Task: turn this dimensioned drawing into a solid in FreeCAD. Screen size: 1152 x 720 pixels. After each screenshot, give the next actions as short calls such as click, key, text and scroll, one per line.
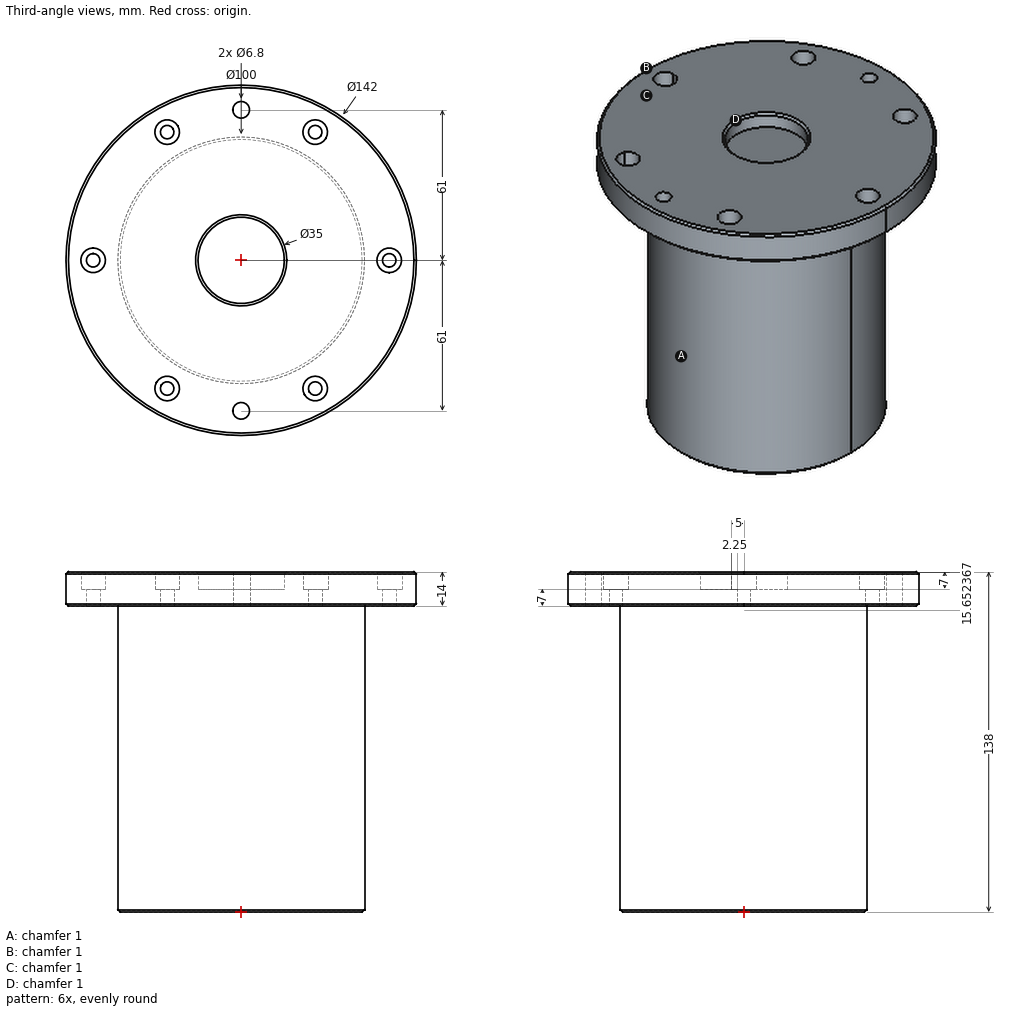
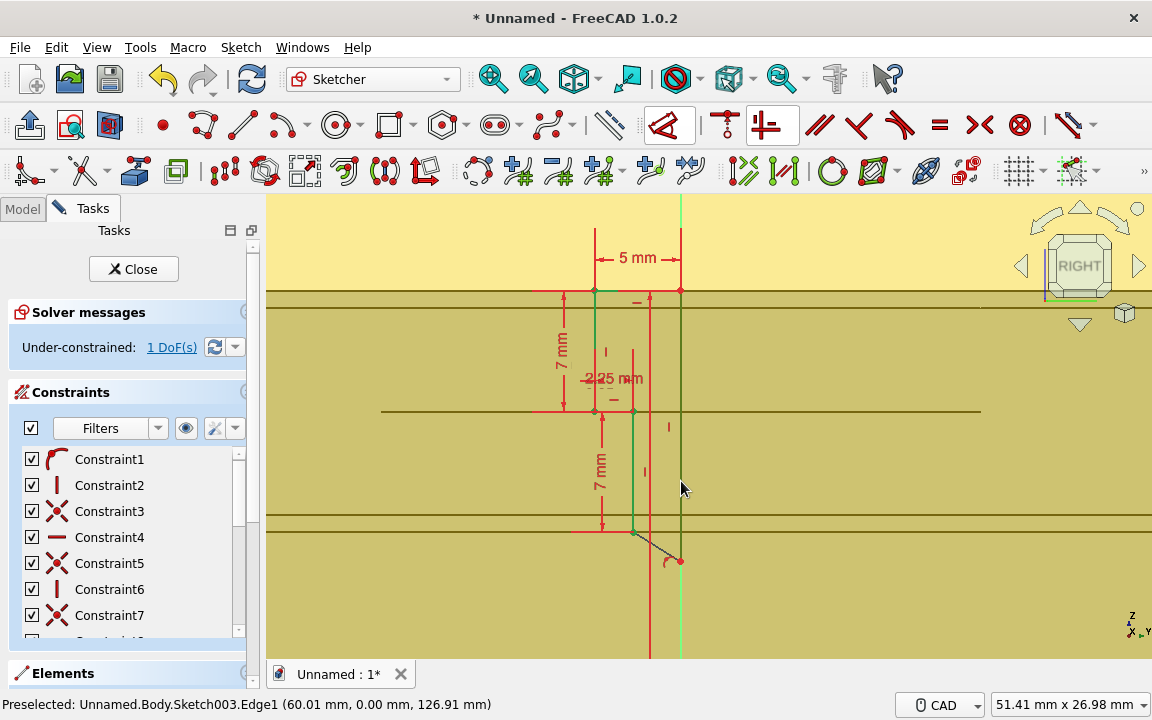
key(i)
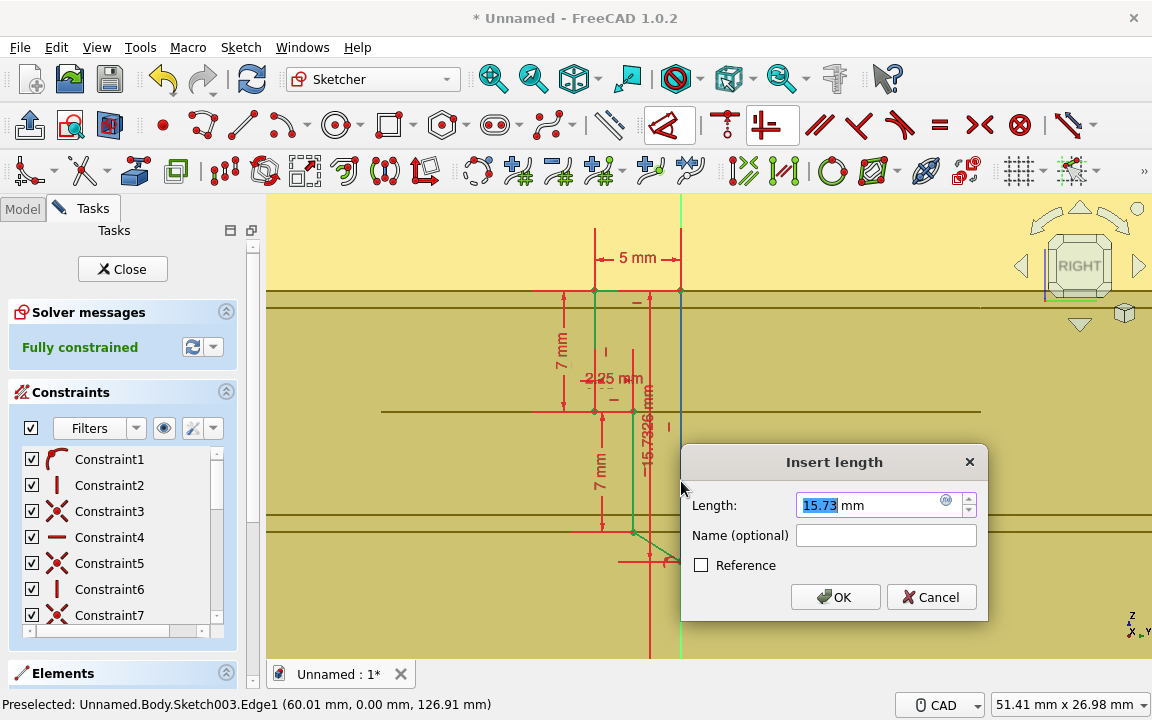
text(15.652367)
key(Return)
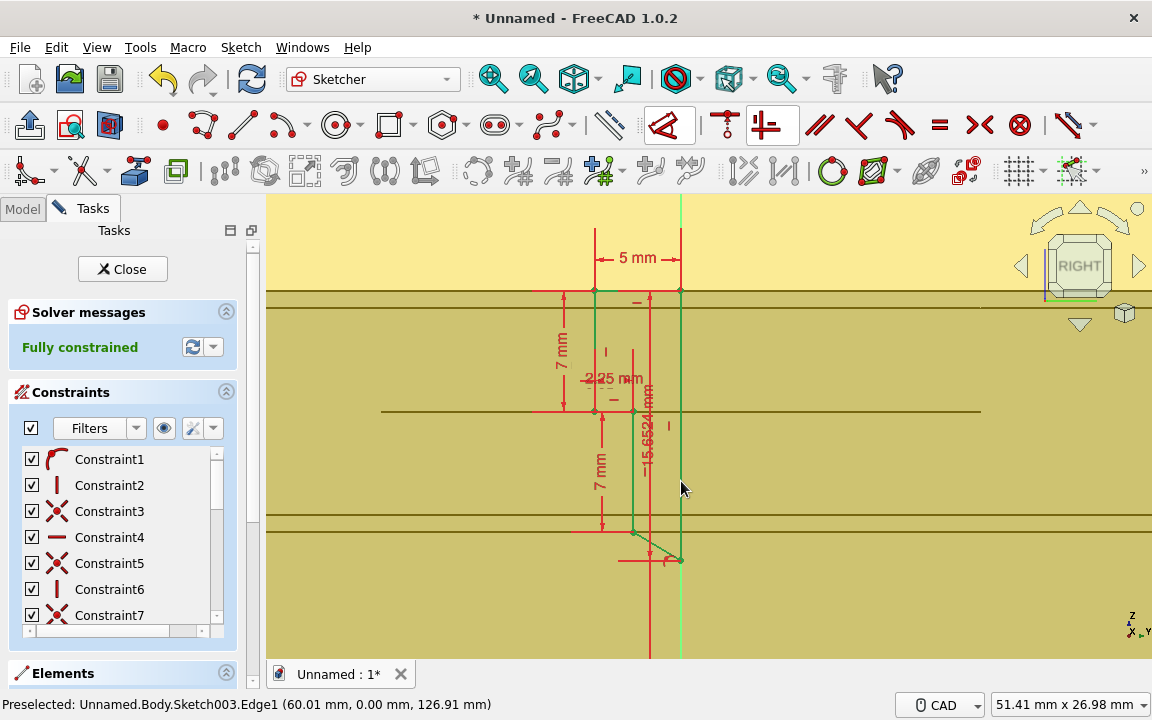
click(123, 269)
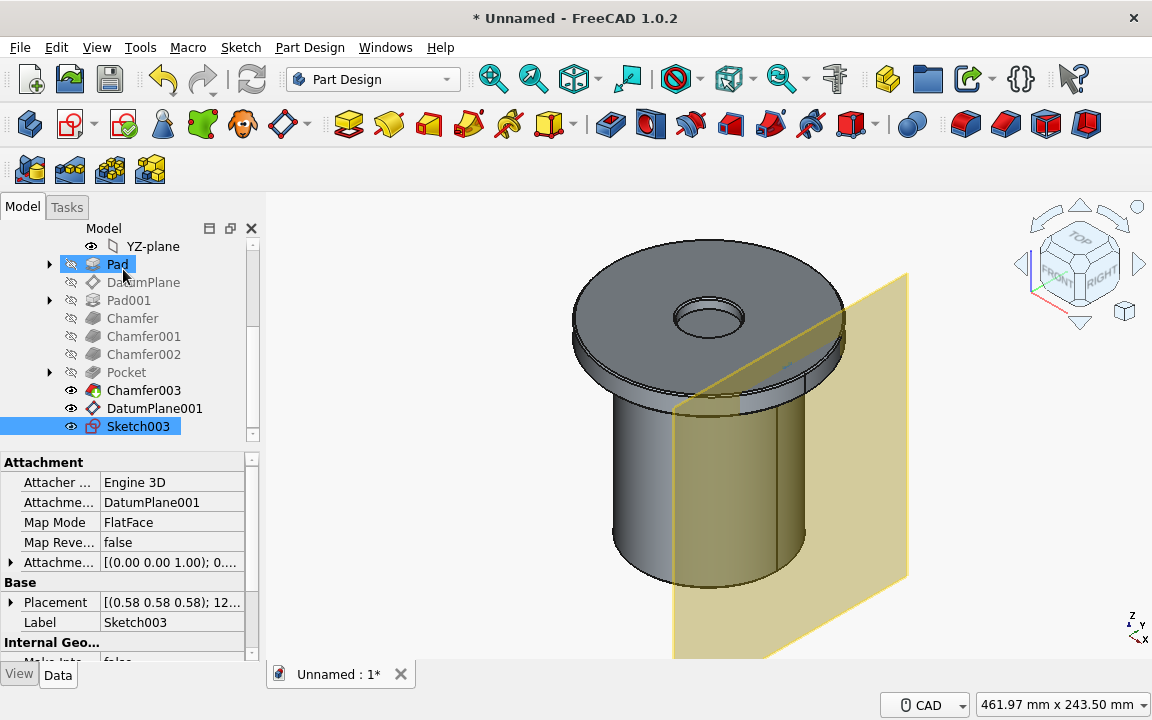
click(692, 124)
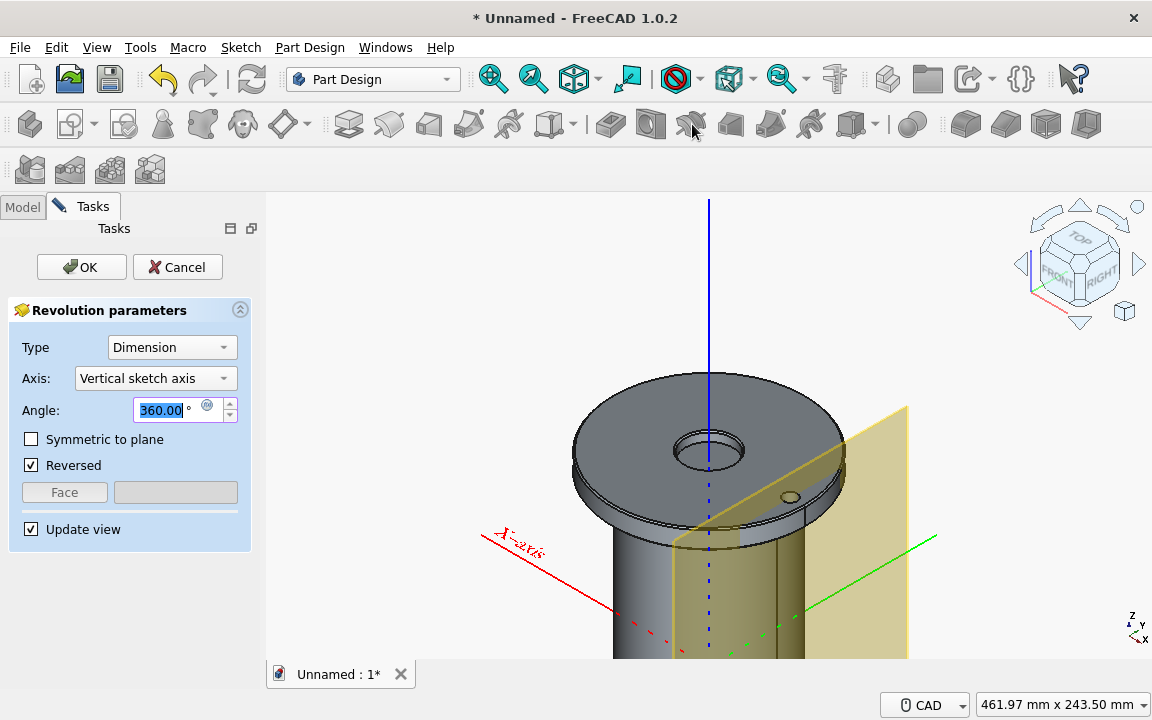
click(82, 267)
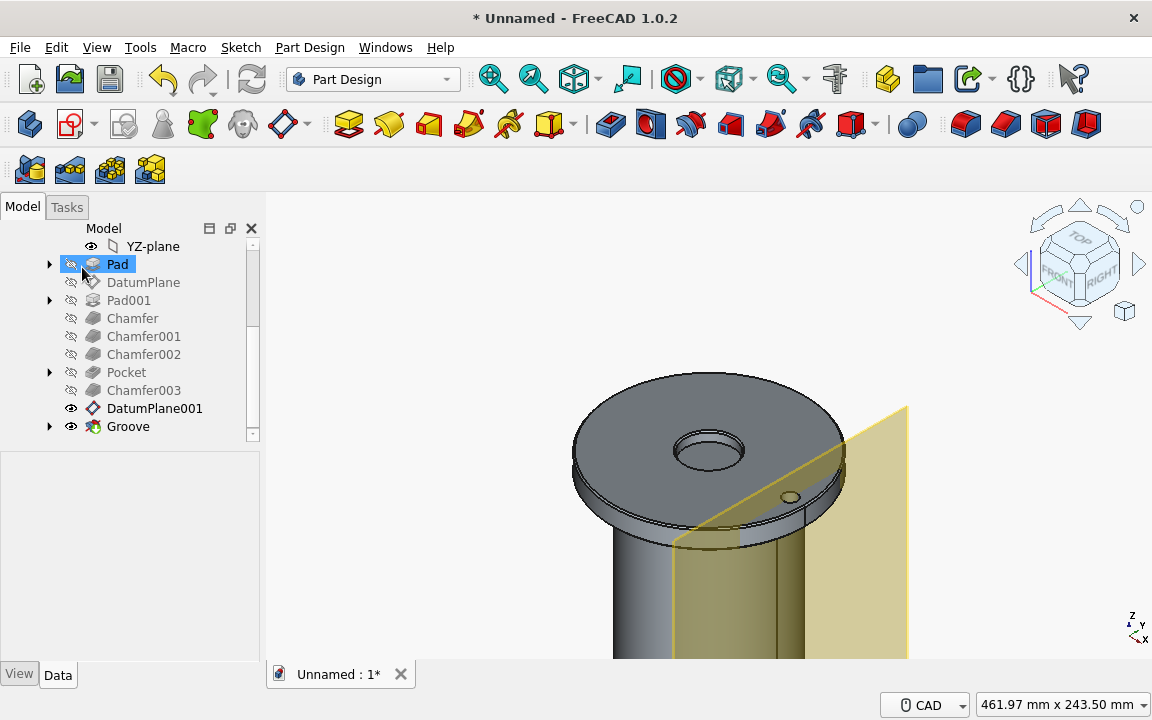
click(116, 408)
key(space)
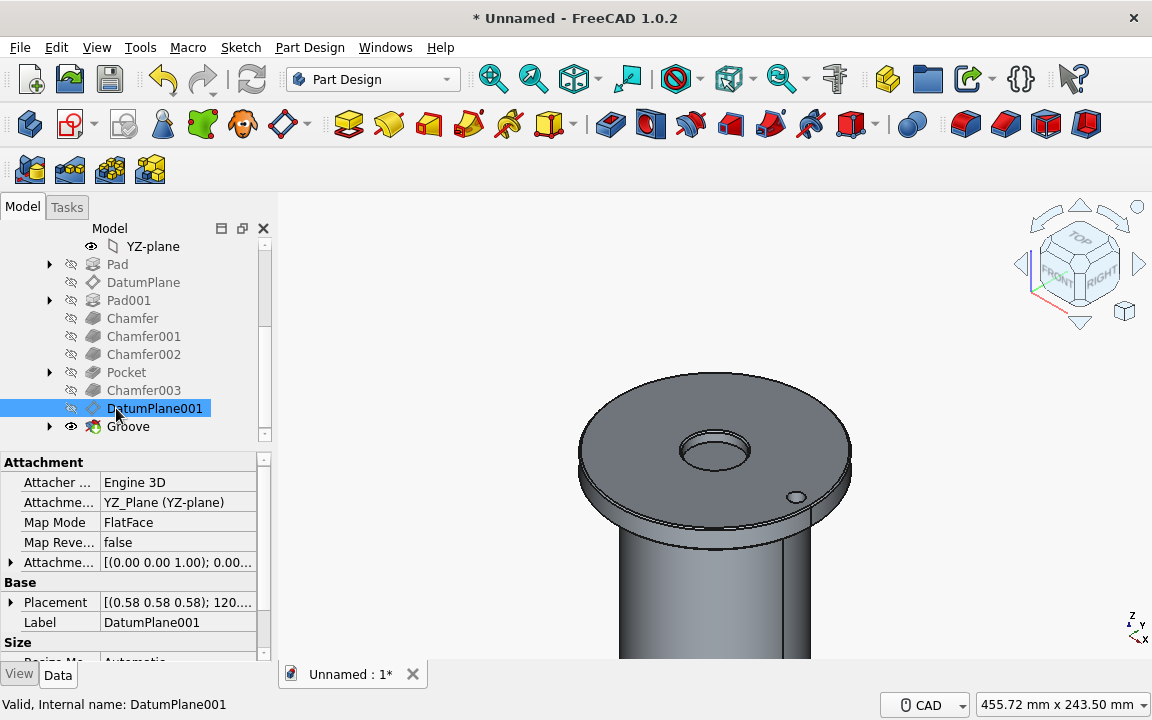
key(v)
key(f)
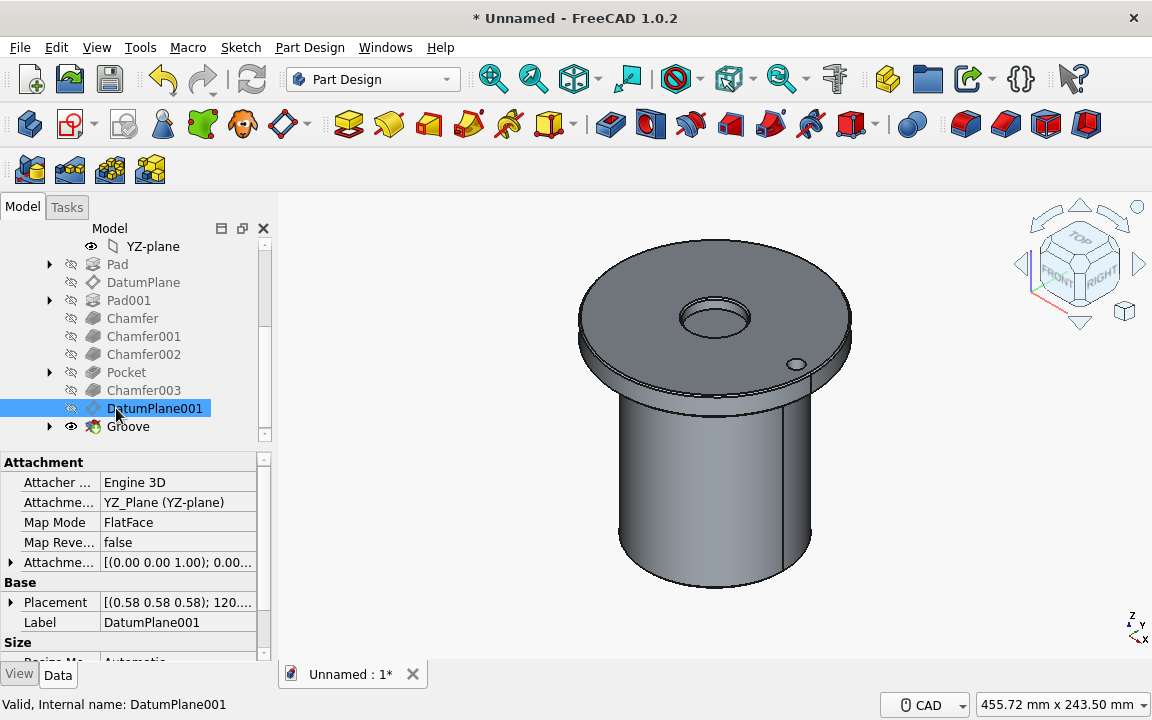
click(116, 426)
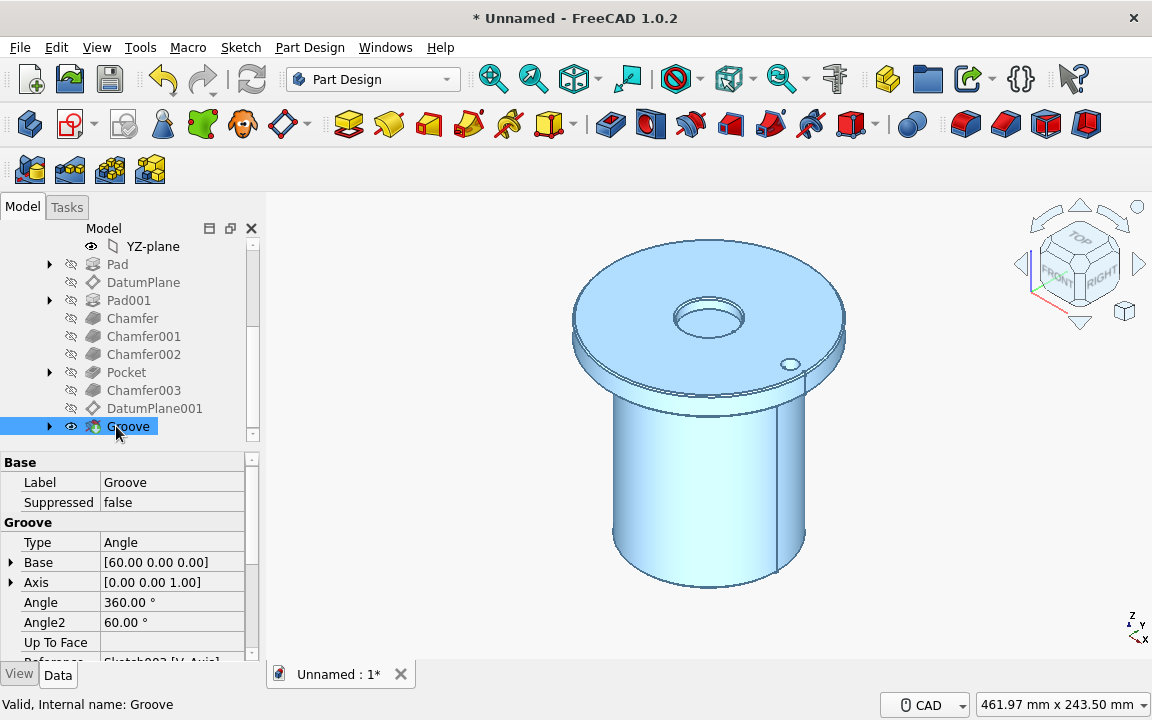
click(110, 170)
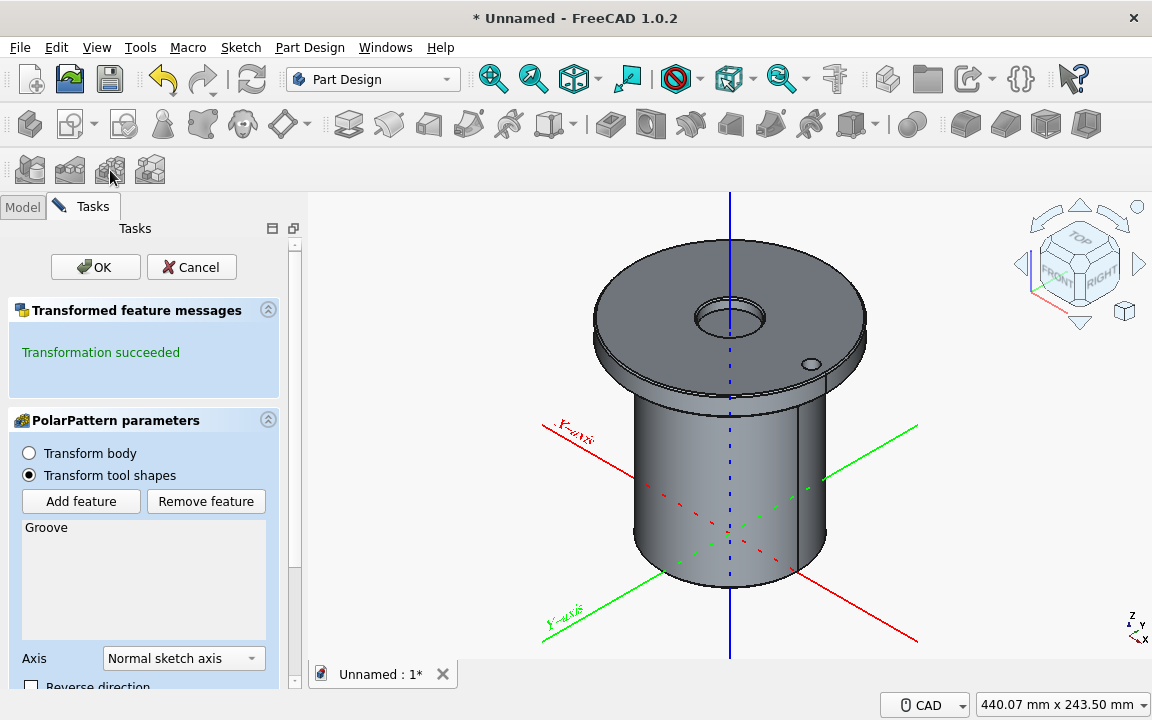
click(184, 658)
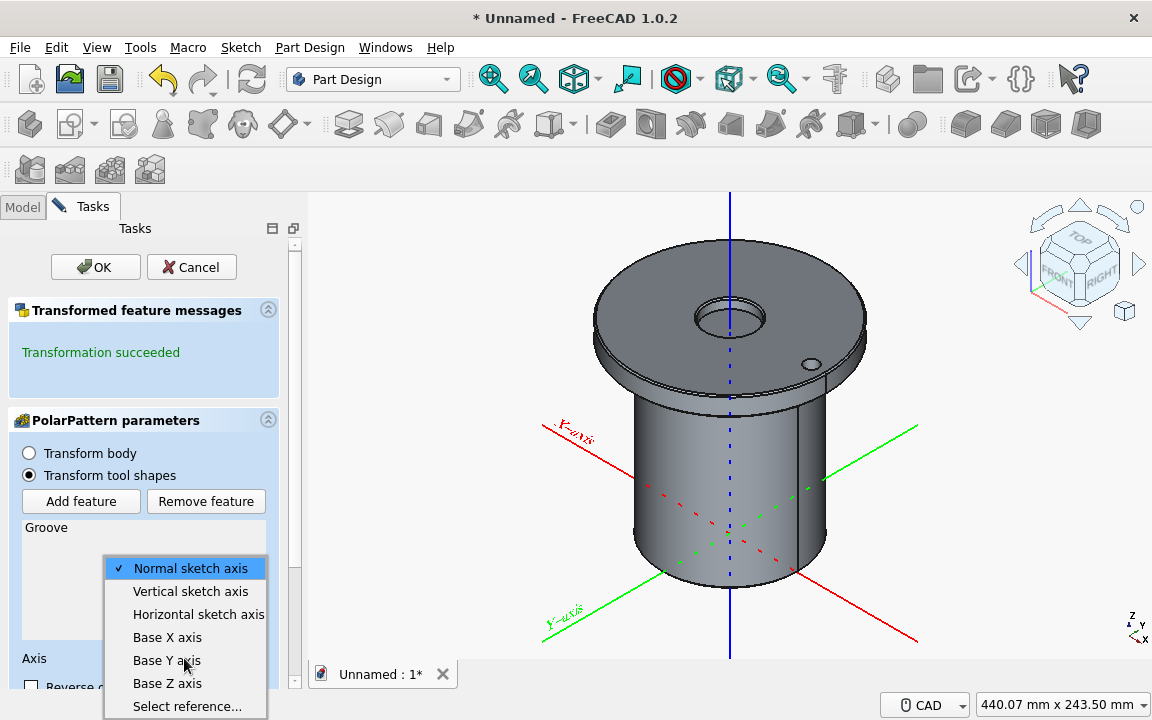
click(184, 684)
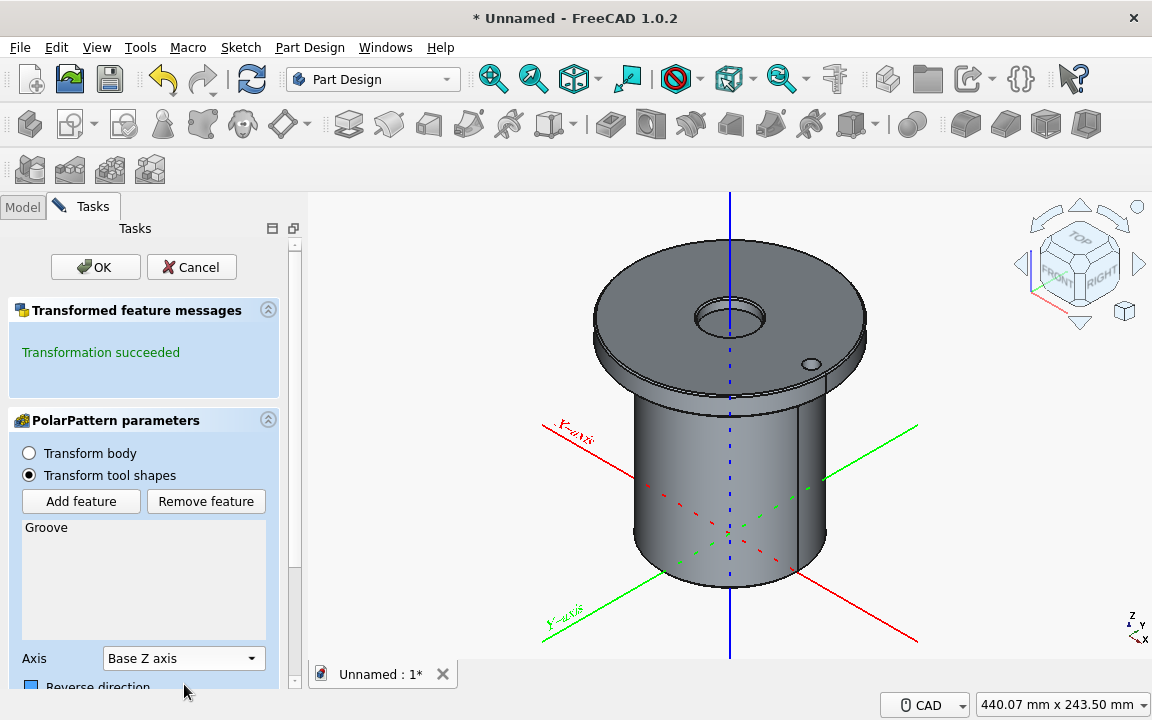
scroll(295, 463, down, 3)